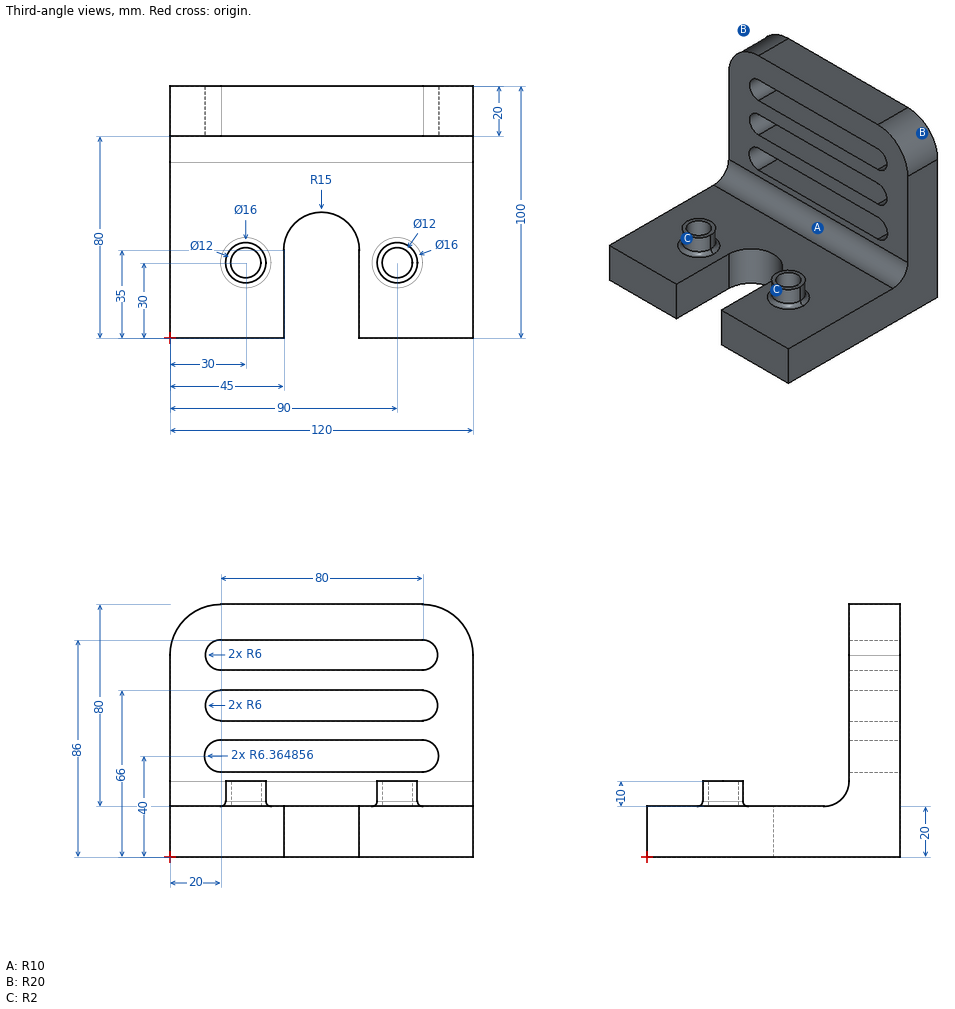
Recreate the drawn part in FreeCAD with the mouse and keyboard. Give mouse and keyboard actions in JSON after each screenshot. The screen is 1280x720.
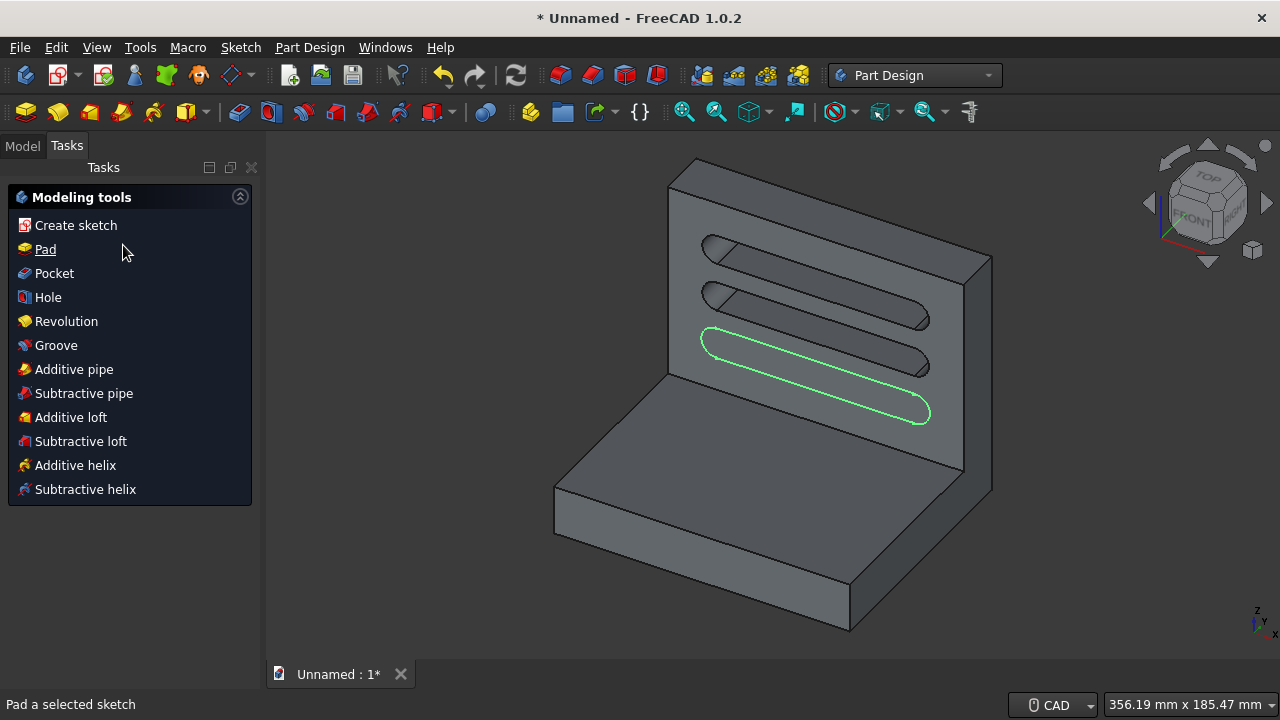
{"action": "left_click", "coordinate": [240, 112]}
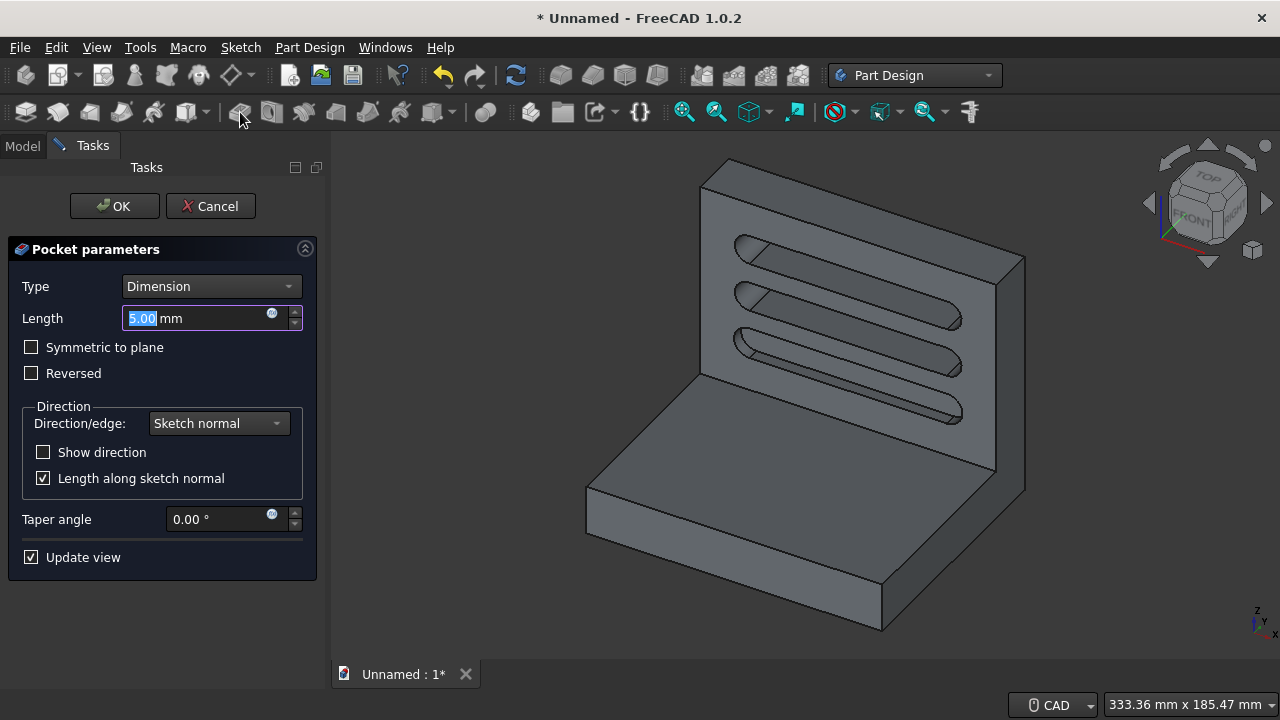
{"action": "left_click", "coordinate": [212, 286]}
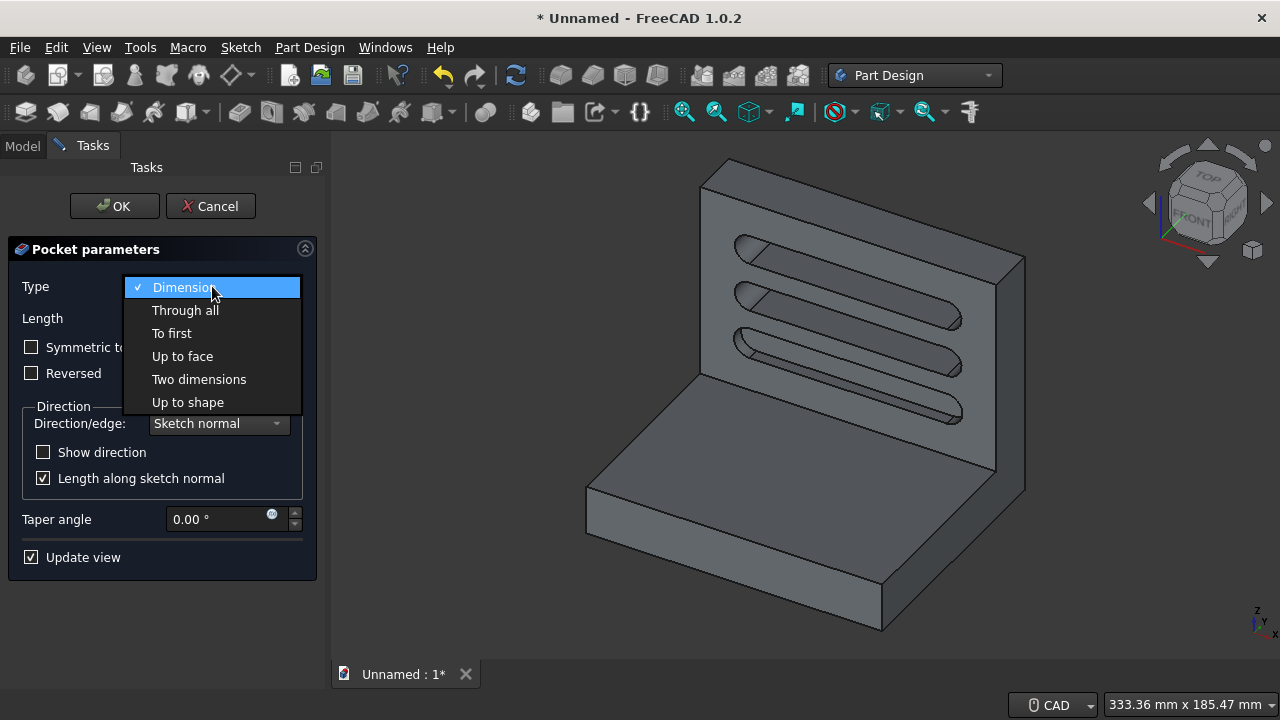
{"action": "left_click", "coordinate": [212, 310]}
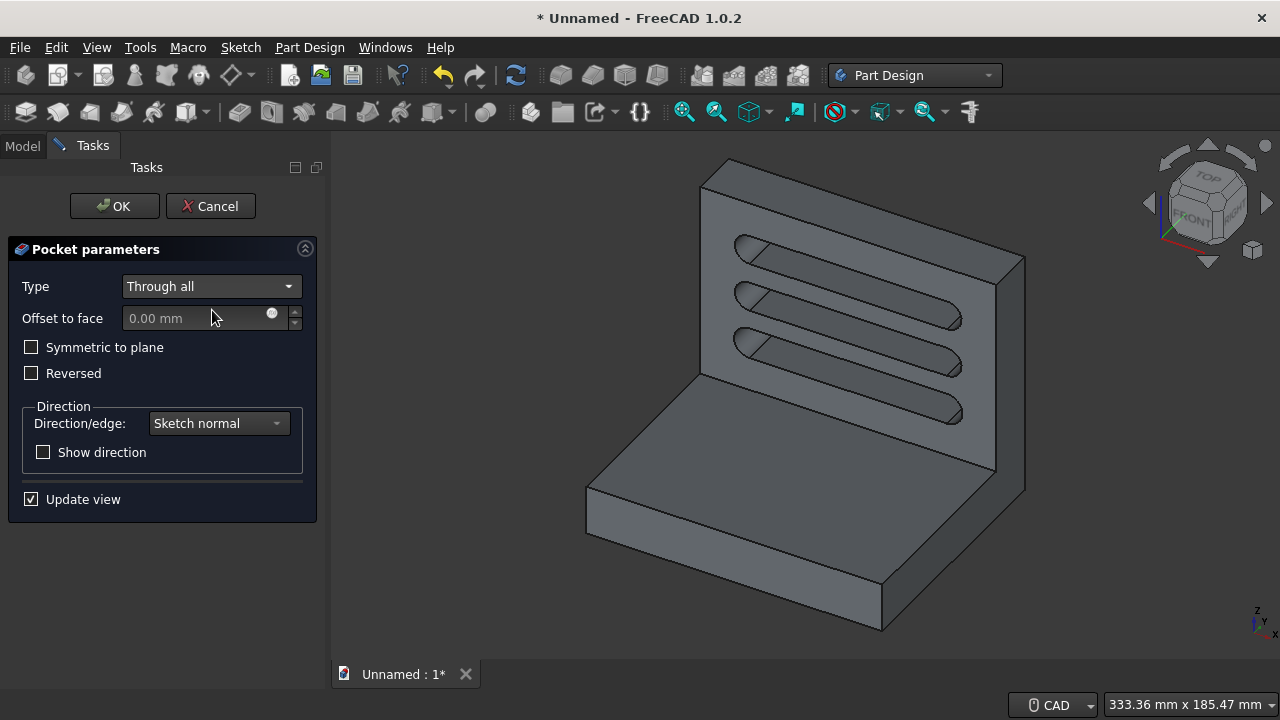
{"action": "left_click", "coordinate": [115, 206]}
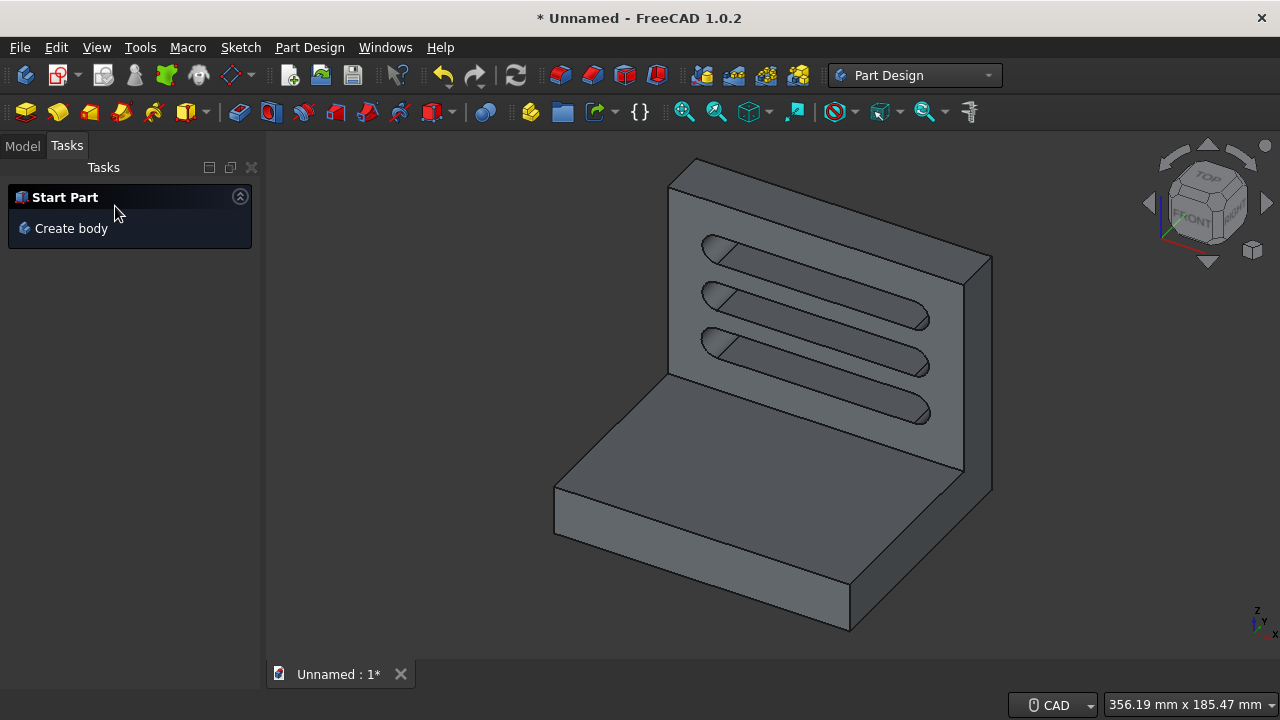
{"action": "key", "text": "0"}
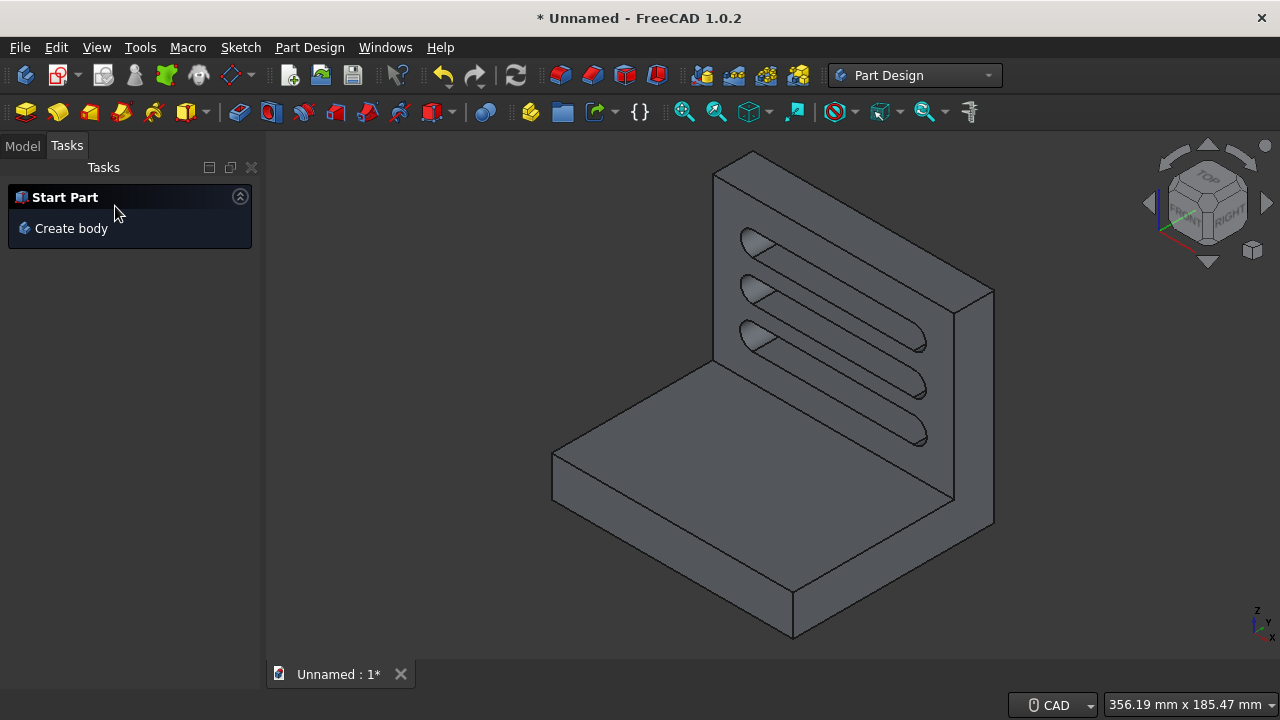
{"action": "key", "text": "2"}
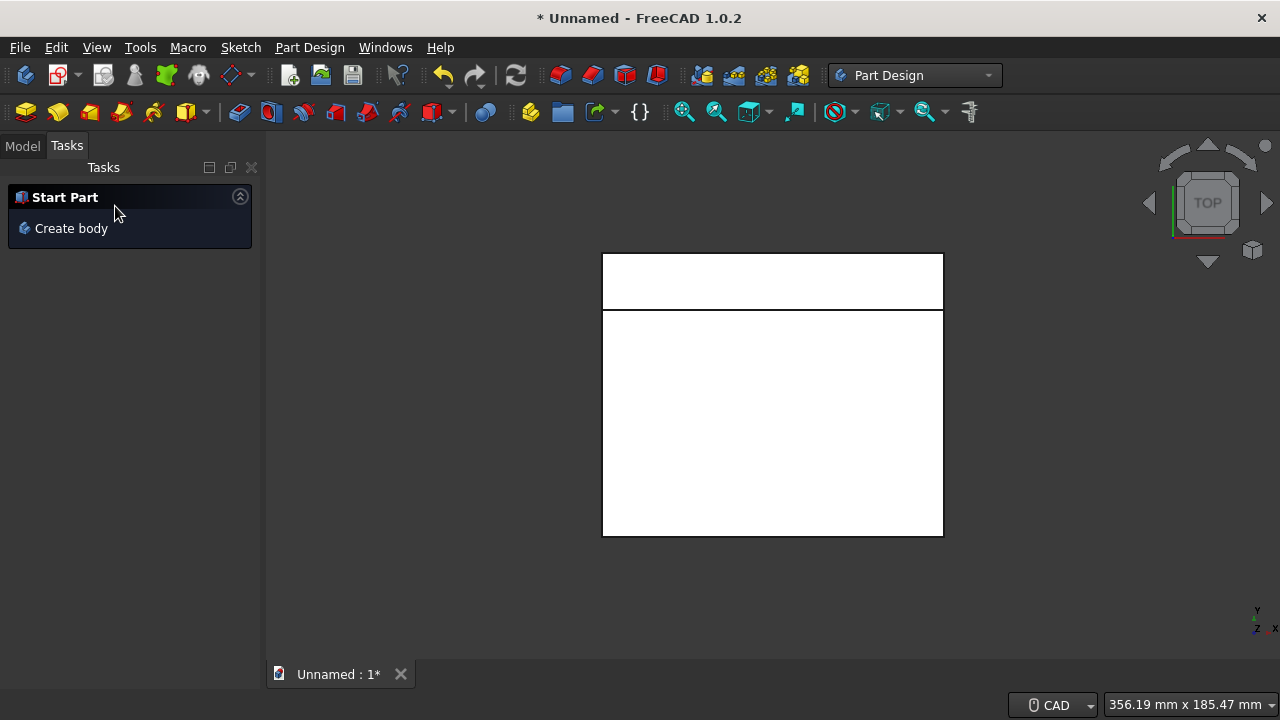
{"action": "key", "text": "1"}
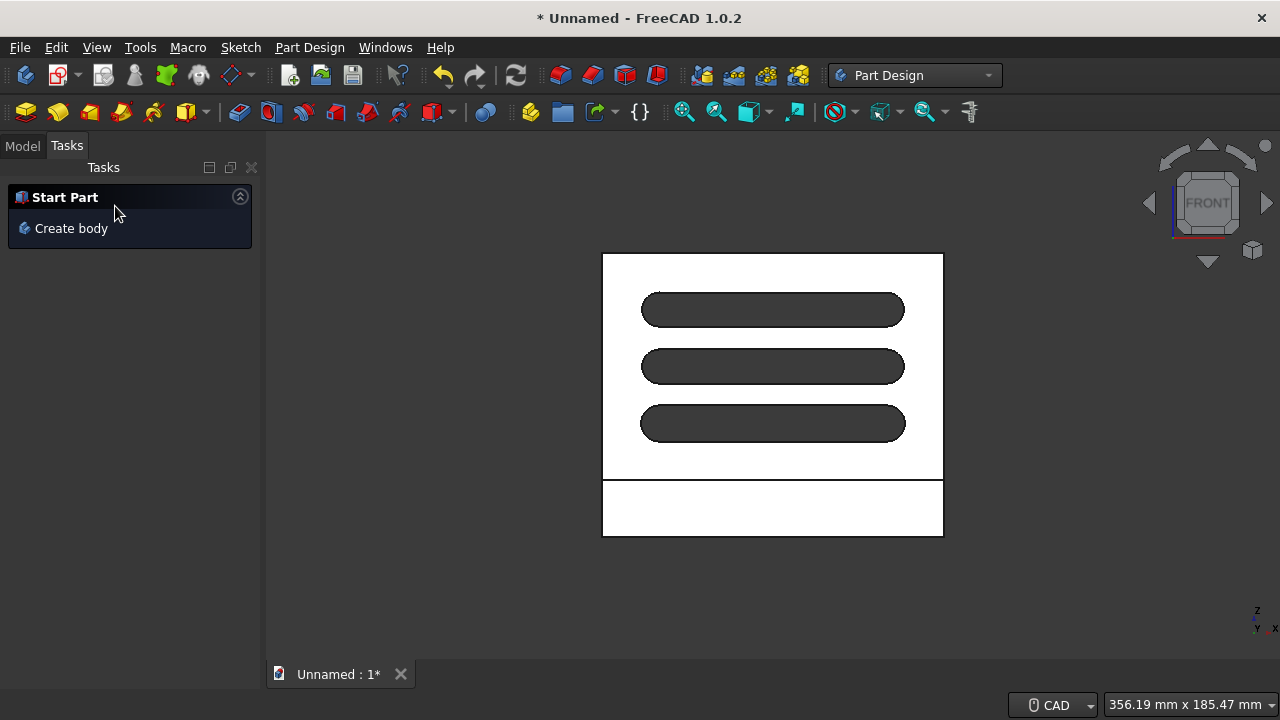
{"action": "key", "text": "3"}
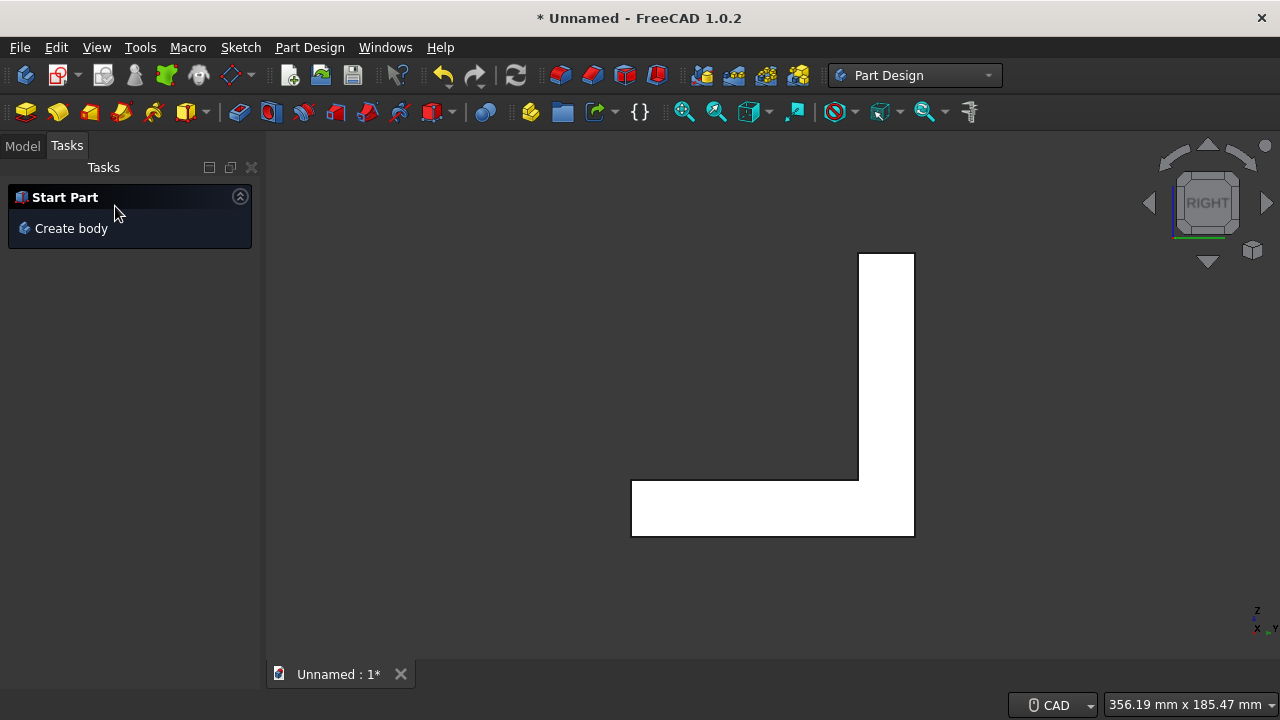
{"action": "key", "text": "5"}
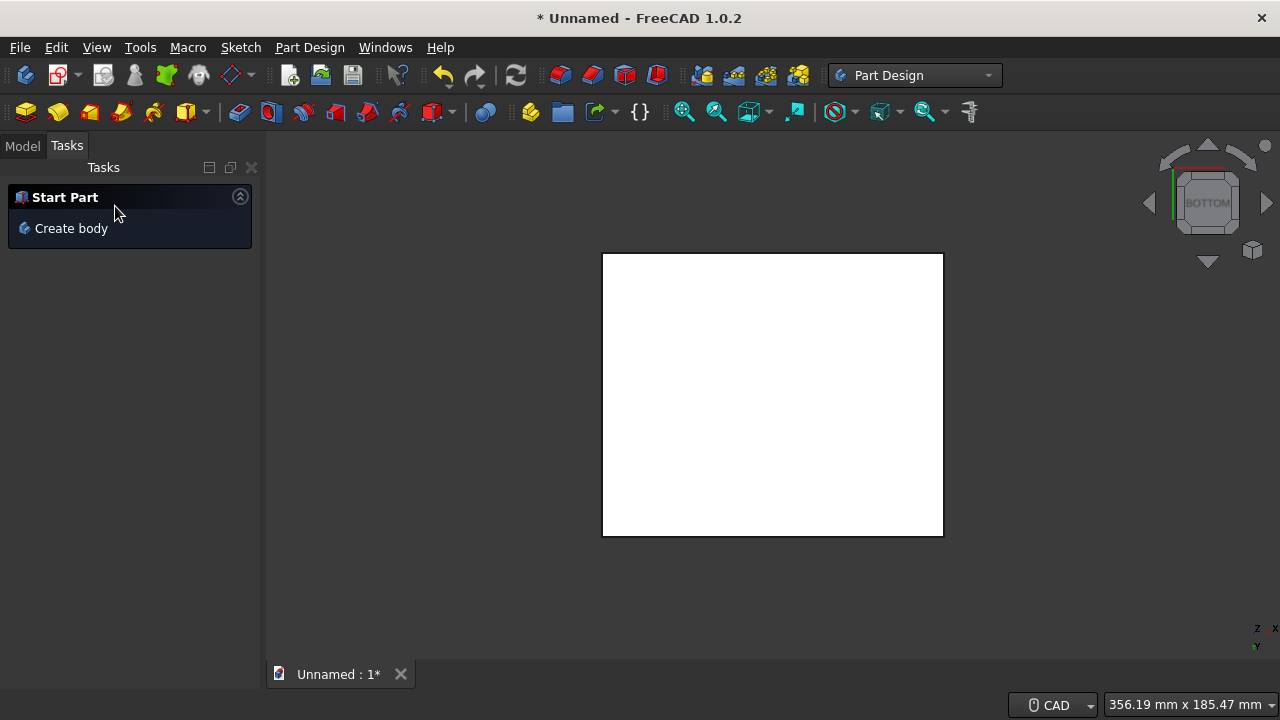
{"action": "key", "text": "4"}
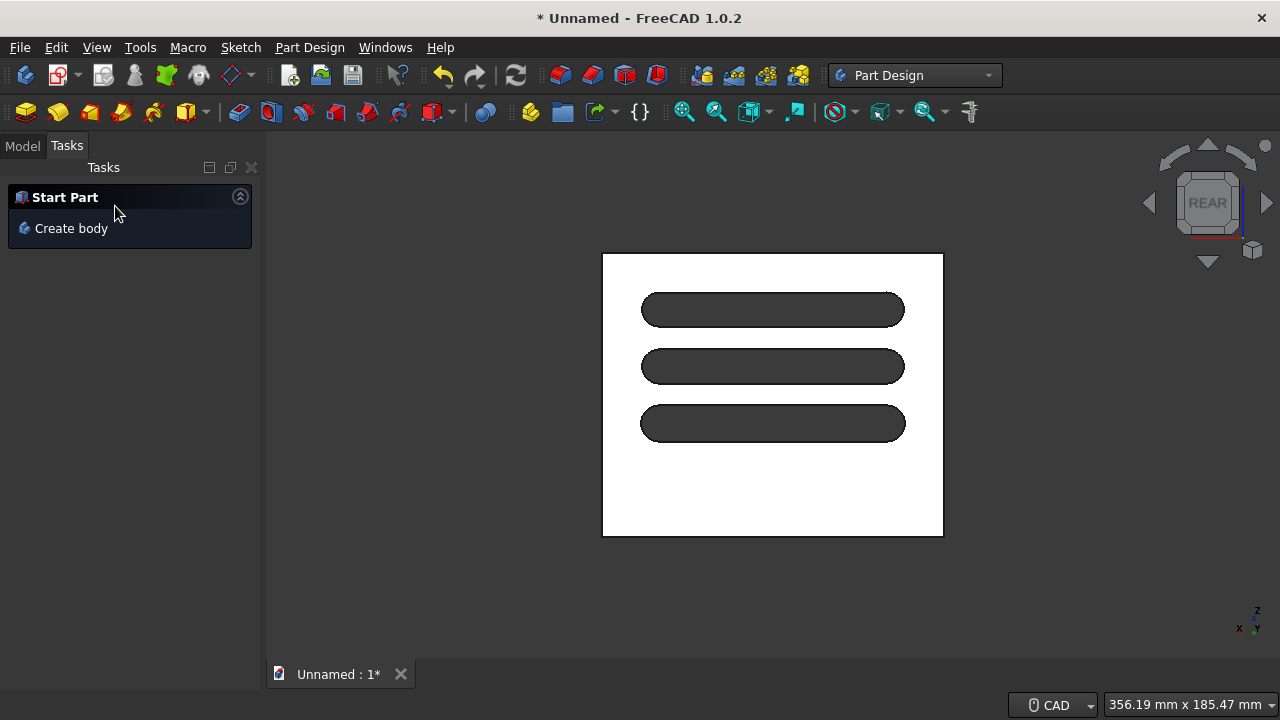
{"action": "key", "text": "6"}